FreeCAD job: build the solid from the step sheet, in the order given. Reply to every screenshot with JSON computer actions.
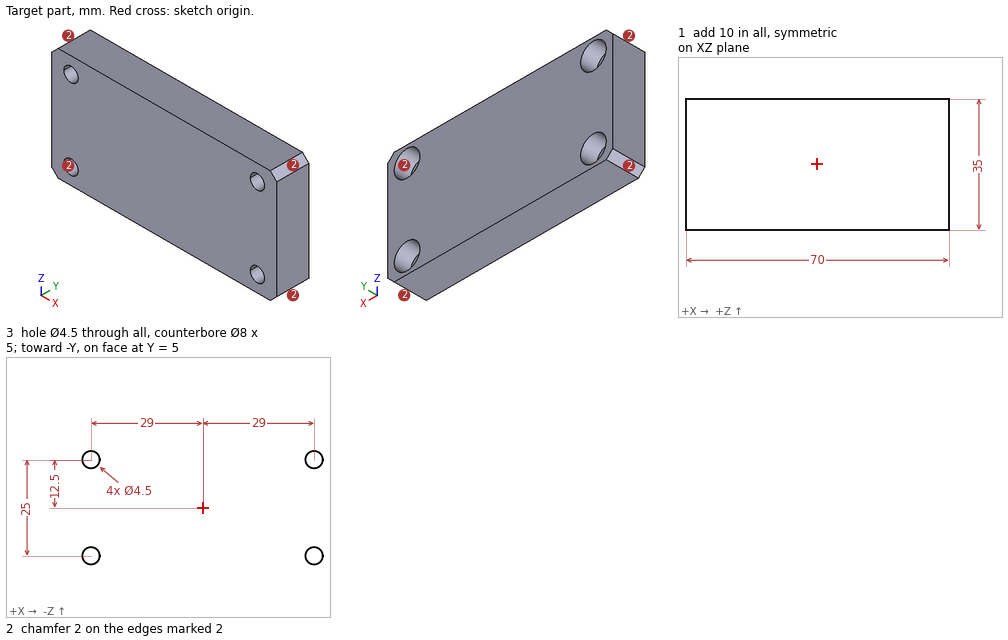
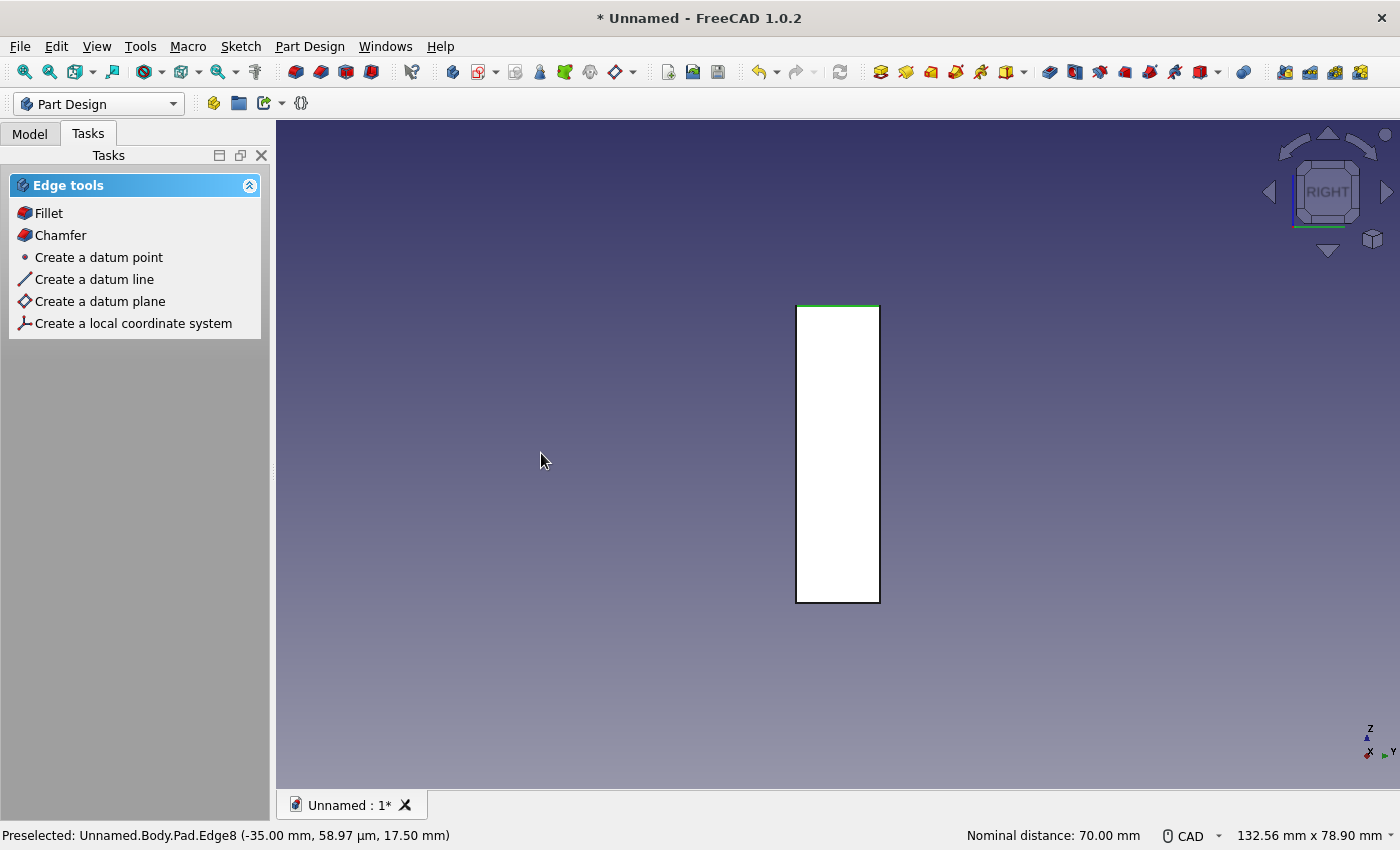
{"action": "left_click", "coordinate": [25, 72]}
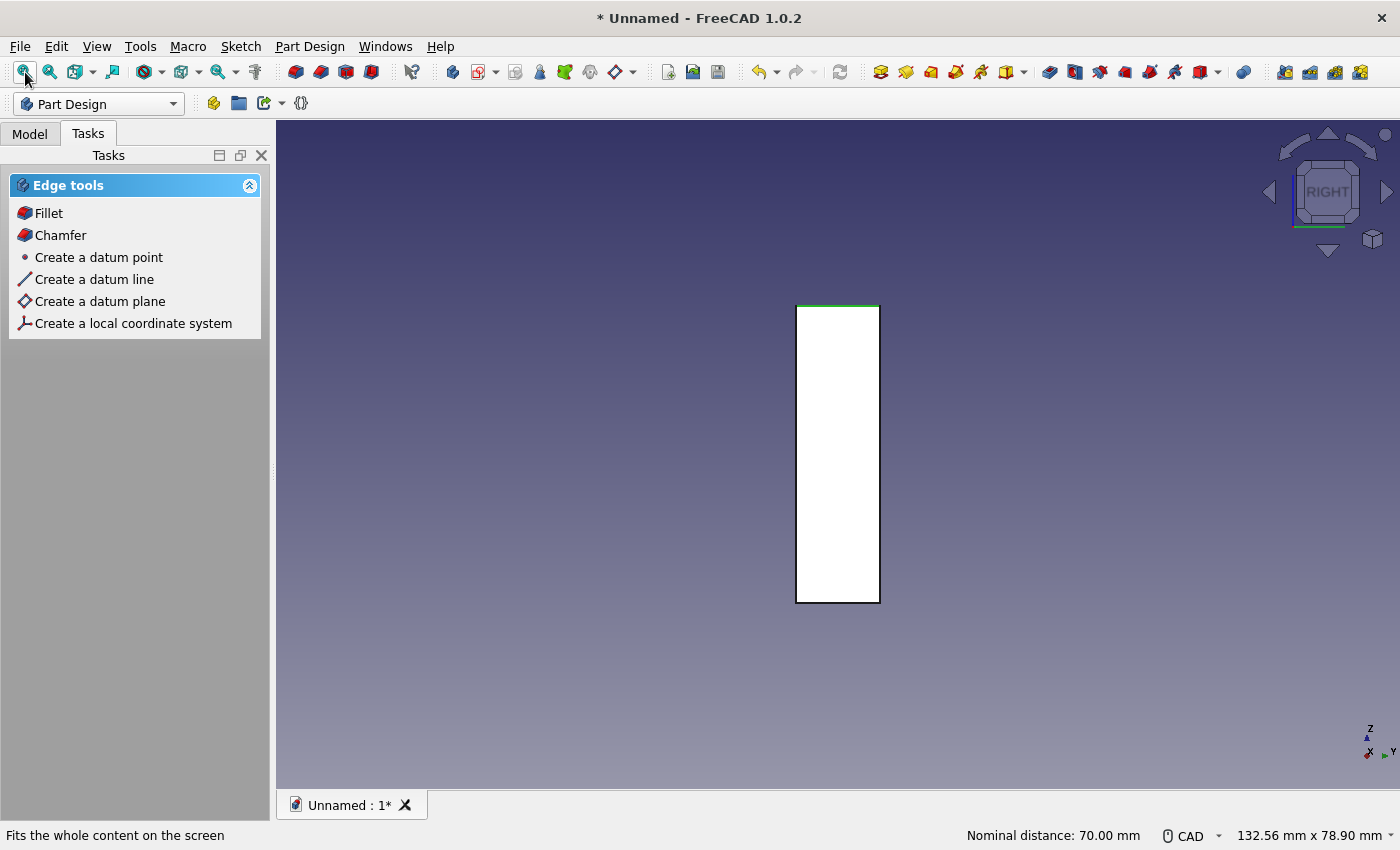
{"action": "left_click", "coordinate": [838, 602], "text": "ctrl"}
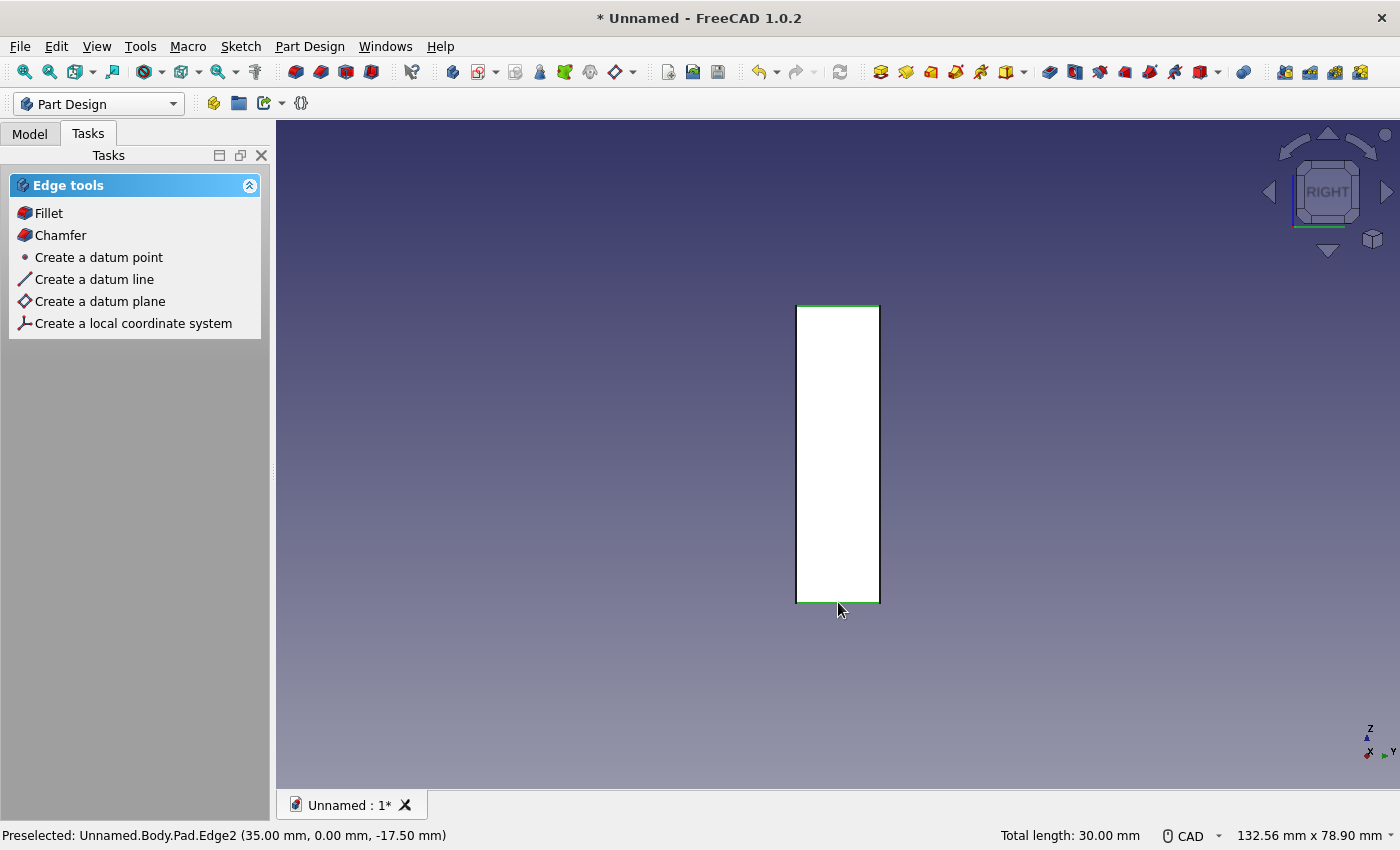
{"action": "key", "text": "5"}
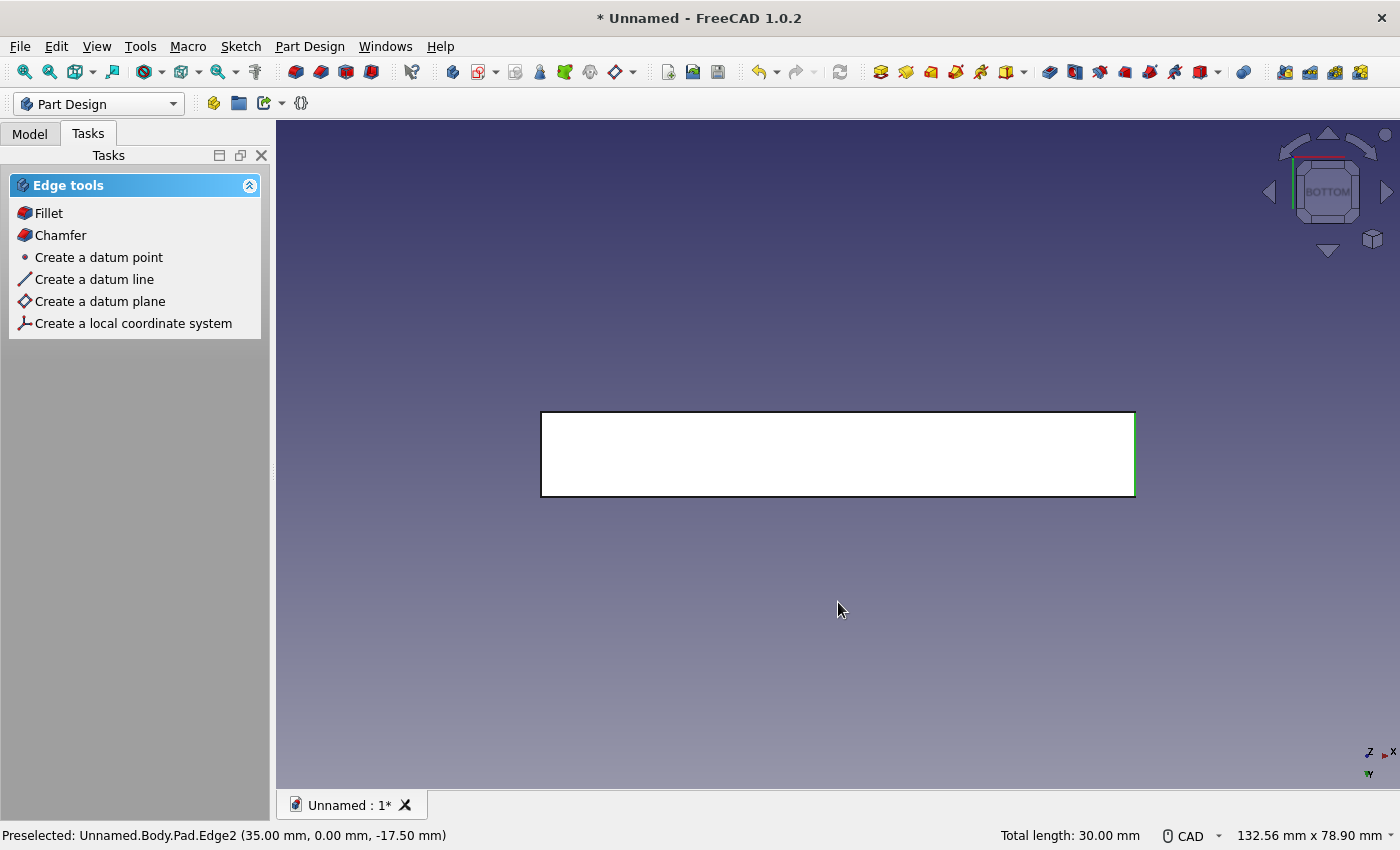
{"action": "left_click", "coordinate": [541, 453], "text": "ctrl"}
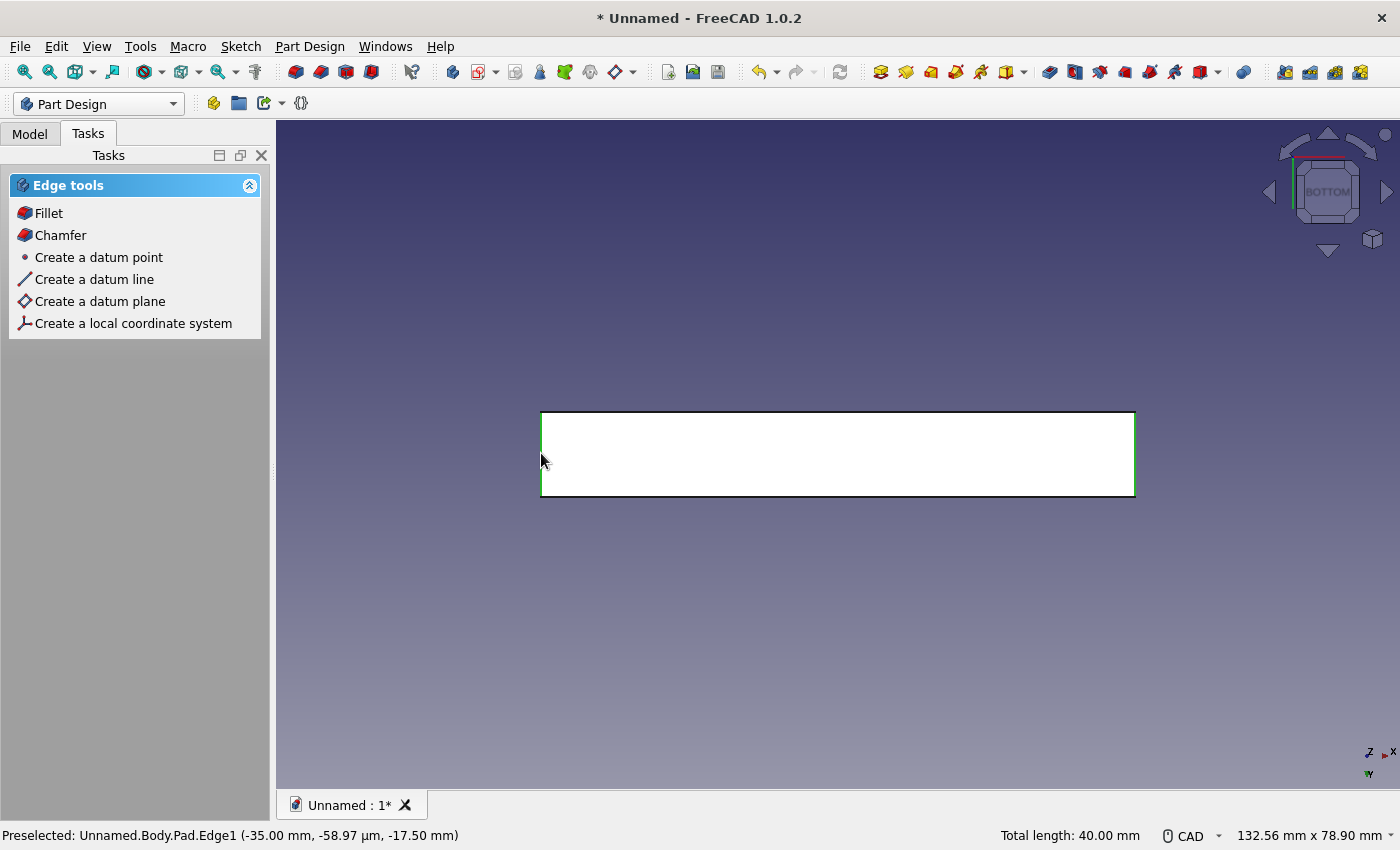
{"action": "left_click", "coordinate": [321, 72]}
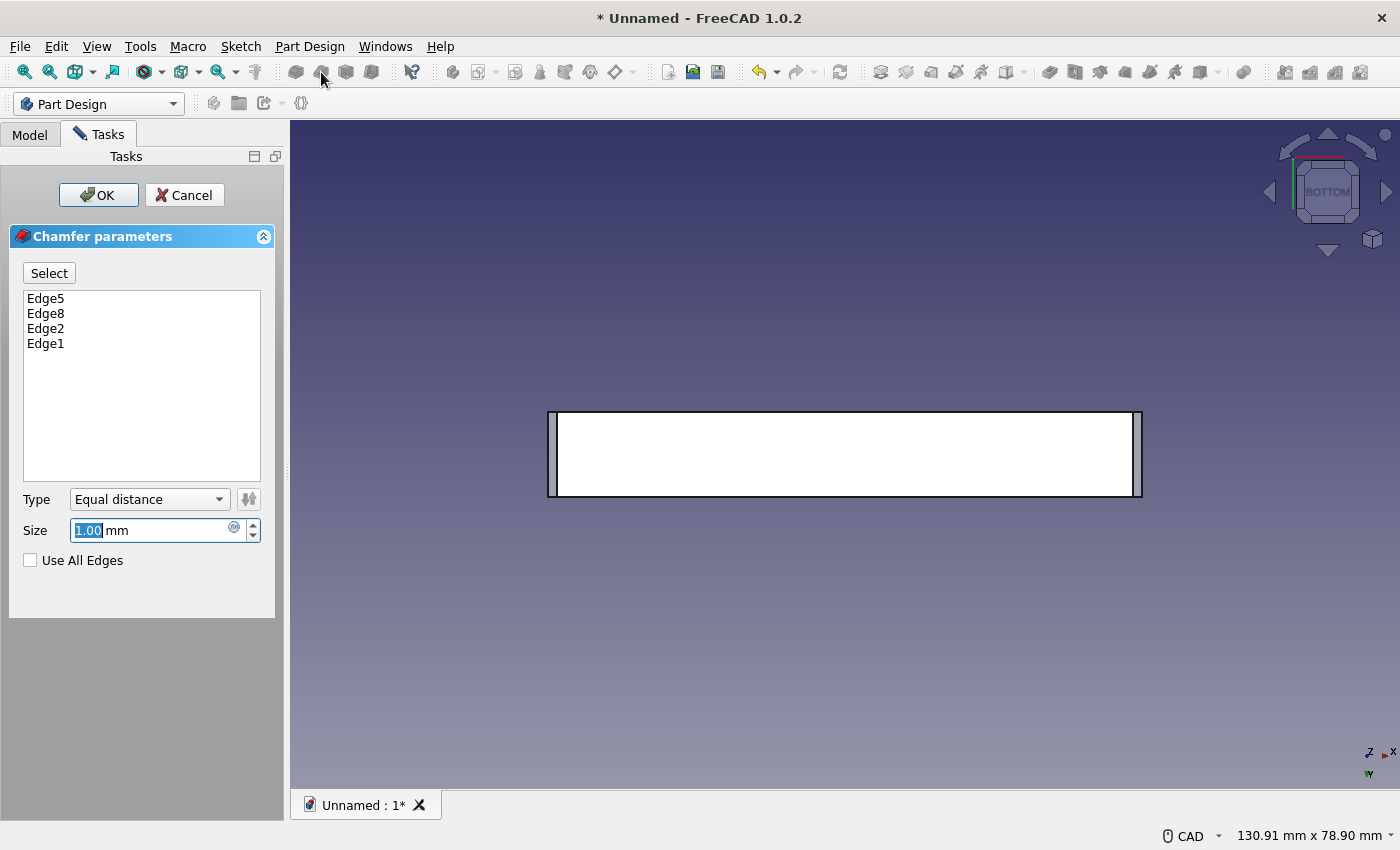
{"action": "type", "text": "2"}
{"action": "key", "text": "Tab"}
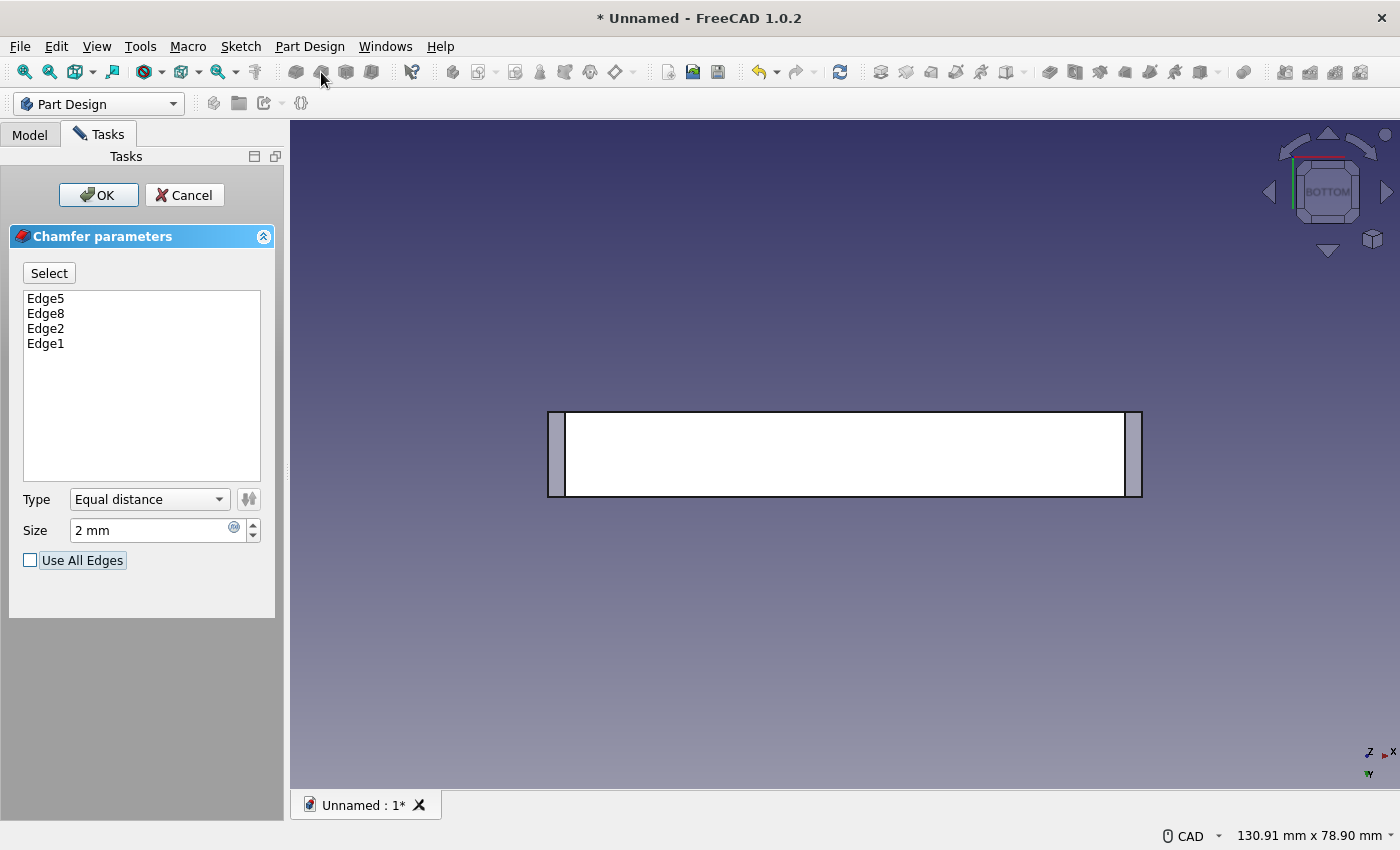
{"action": "left_click", "coordinate": [99, 195]}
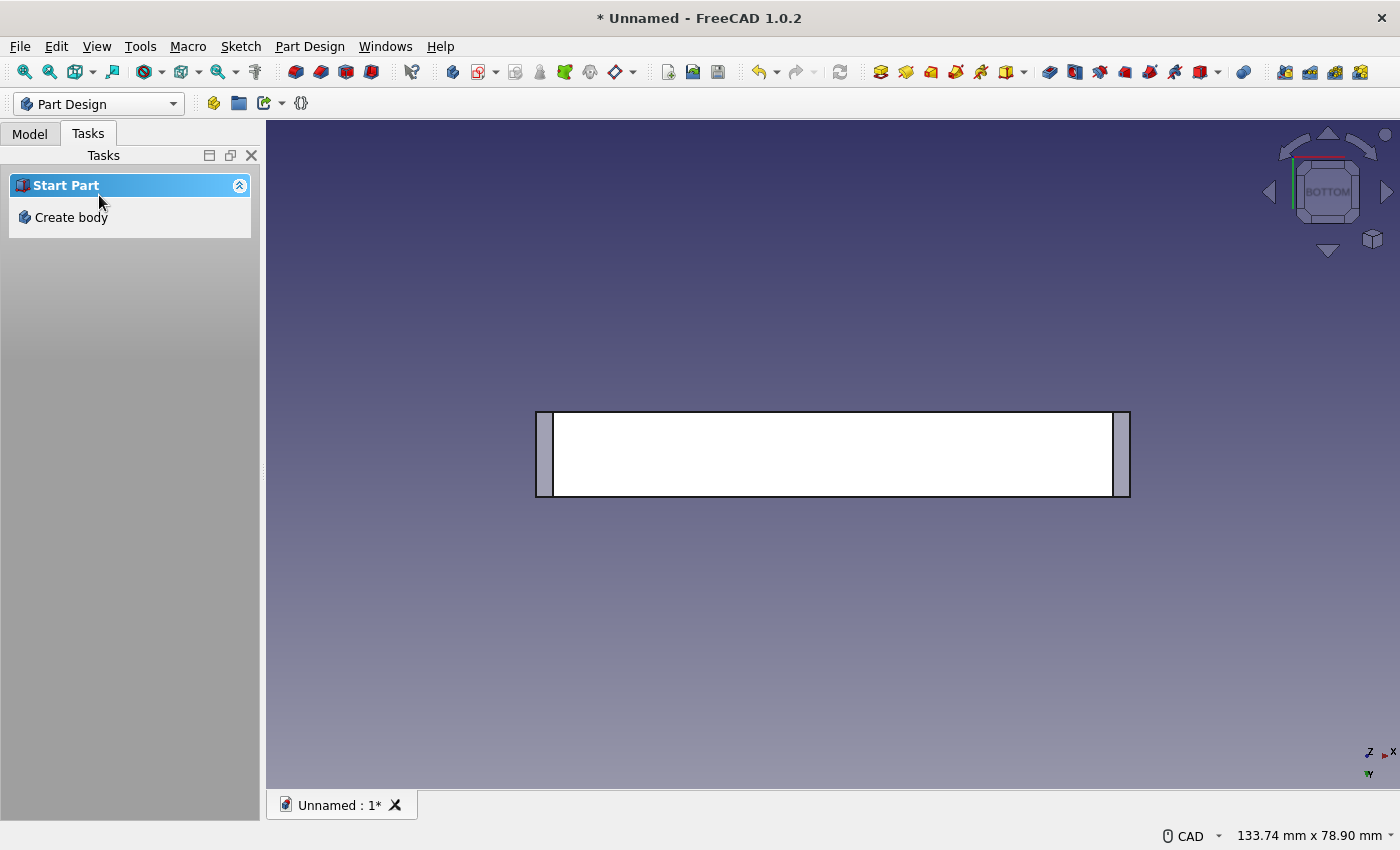
{"action": "key", "text": "4"}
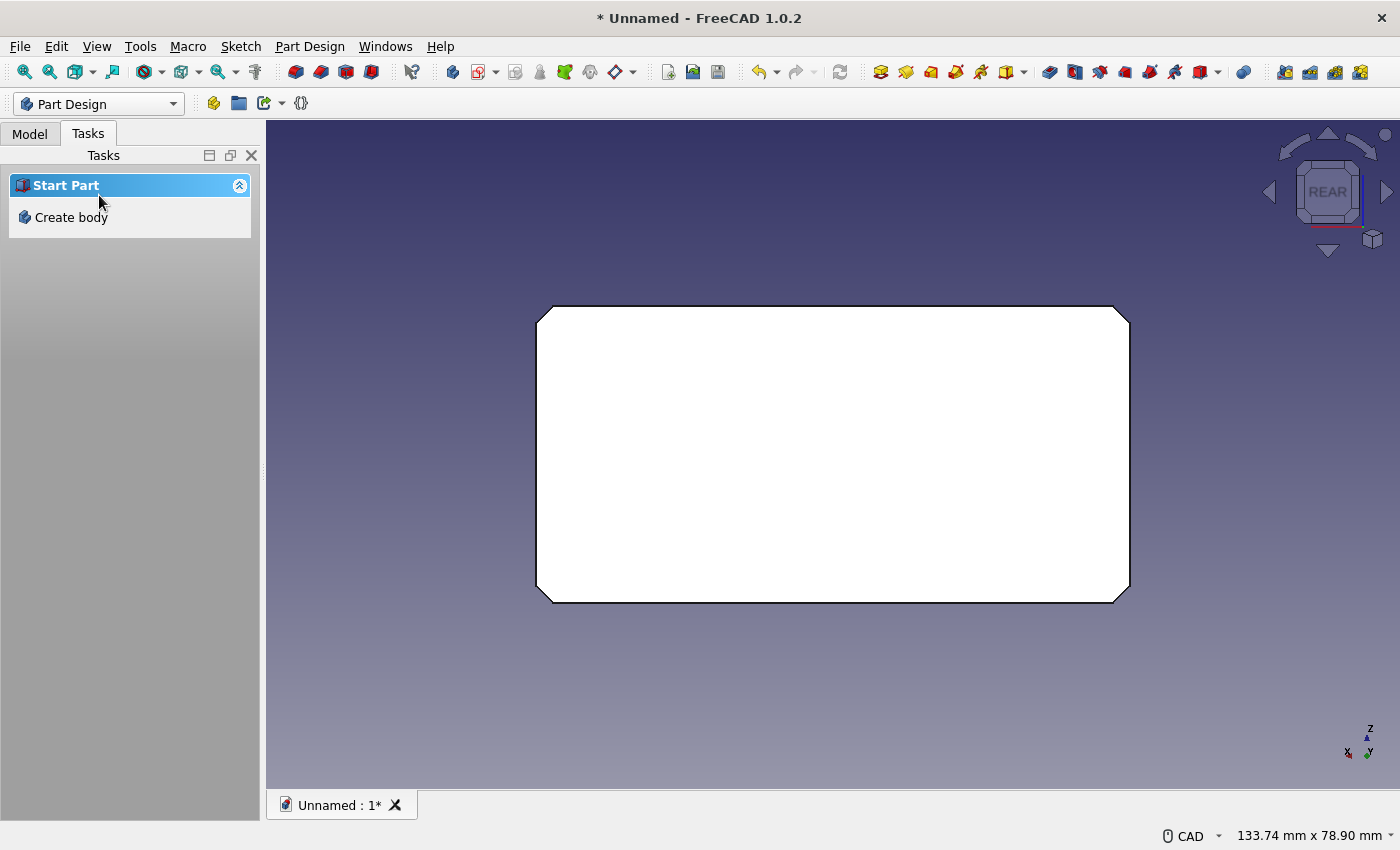
{"action": "left_click", "coordinate": [748, 454]}